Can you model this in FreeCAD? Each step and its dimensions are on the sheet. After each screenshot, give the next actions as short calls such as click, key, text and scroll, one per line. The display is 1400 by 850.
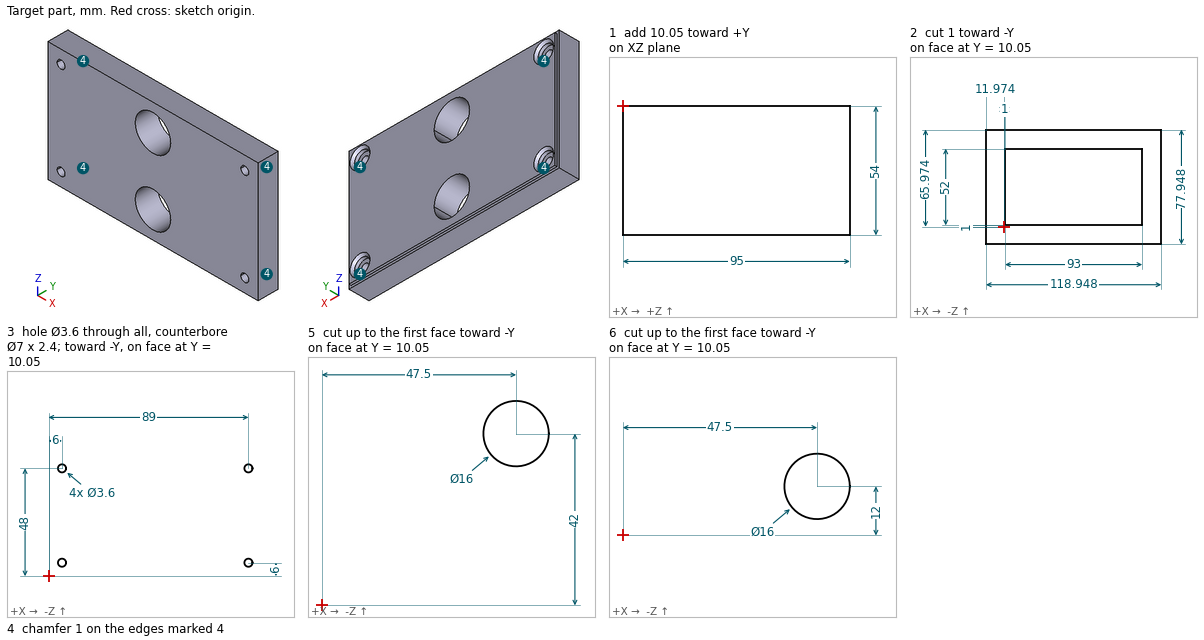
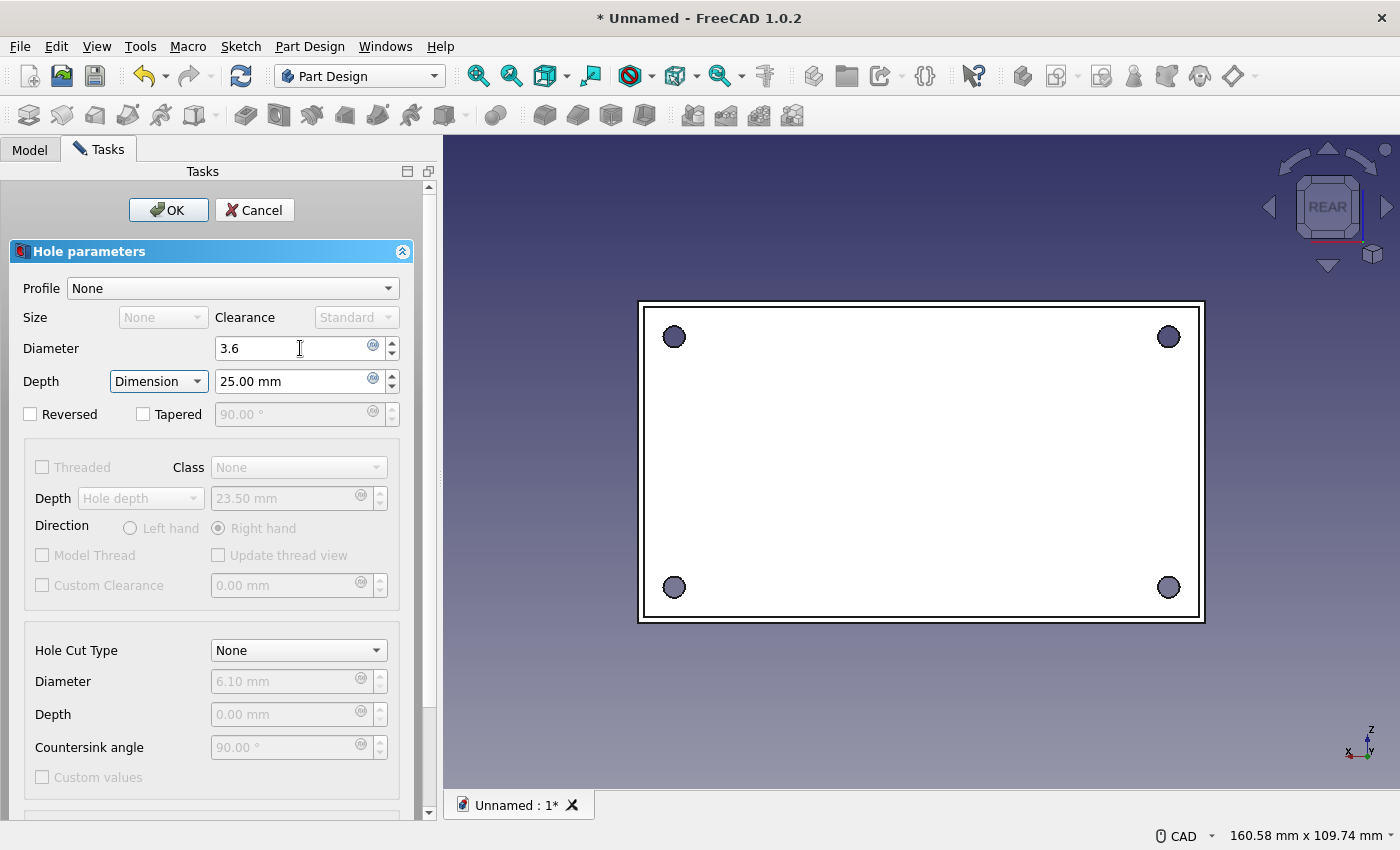
click(160, 382)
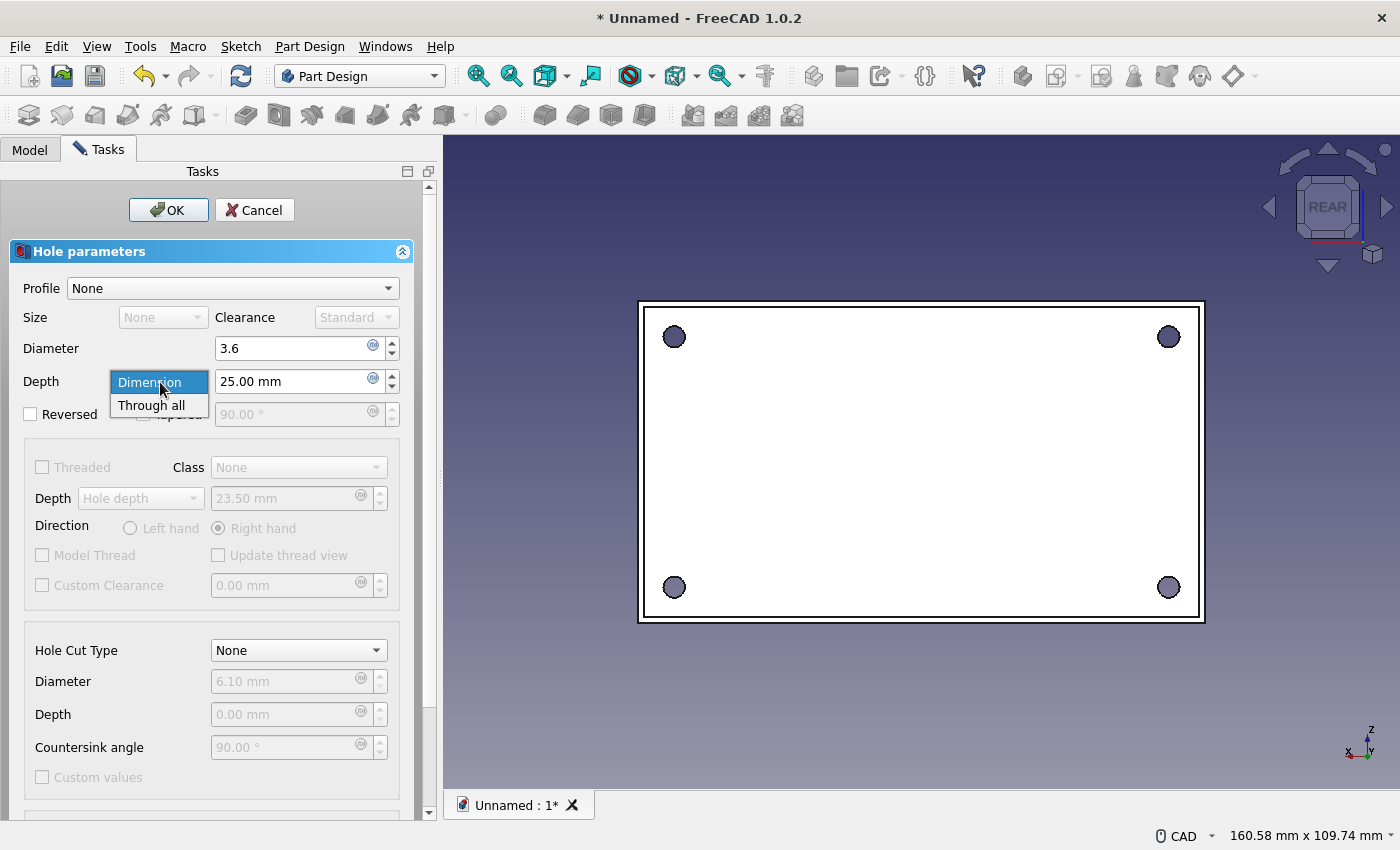
click(158, 406)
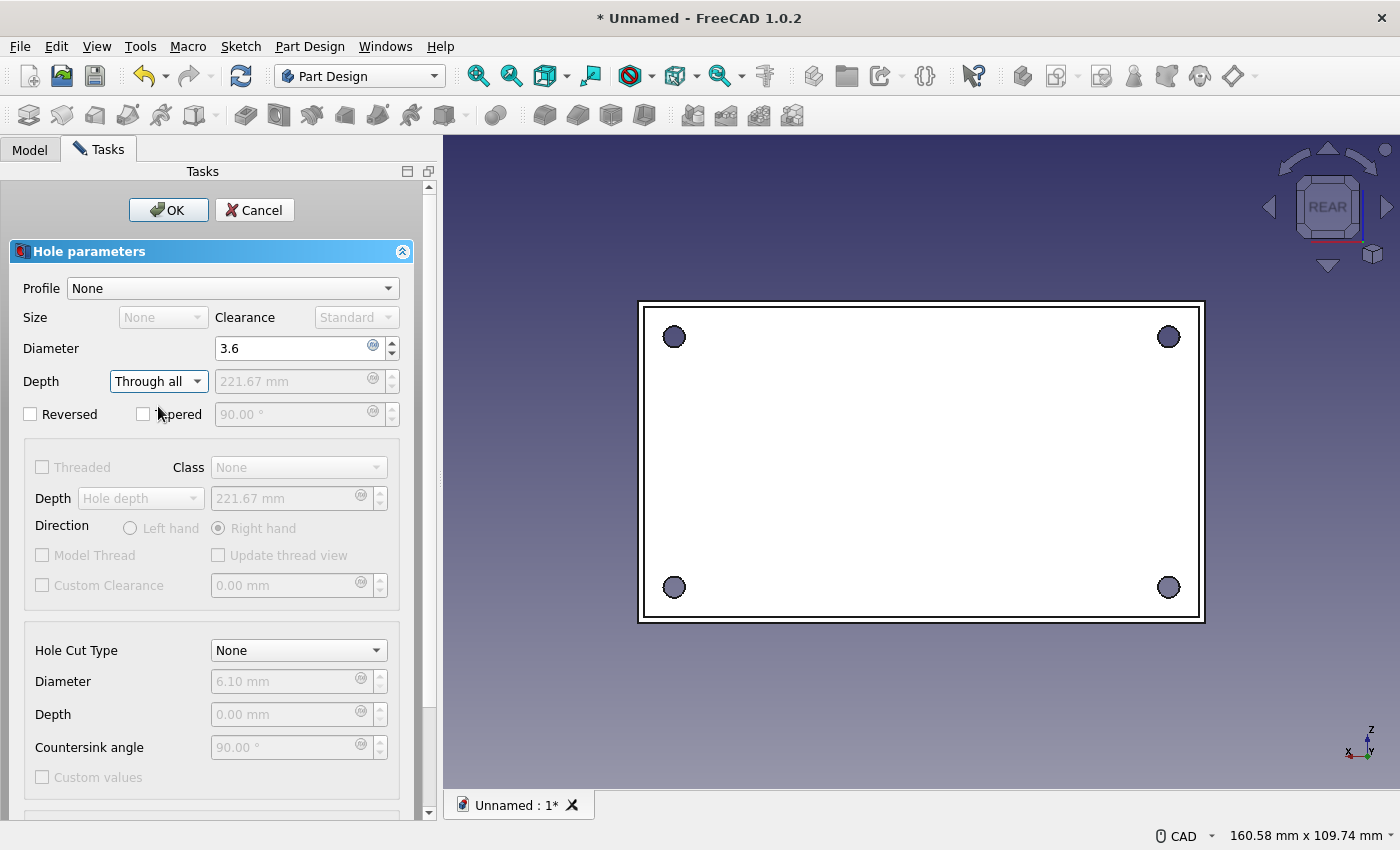
click(300, 650)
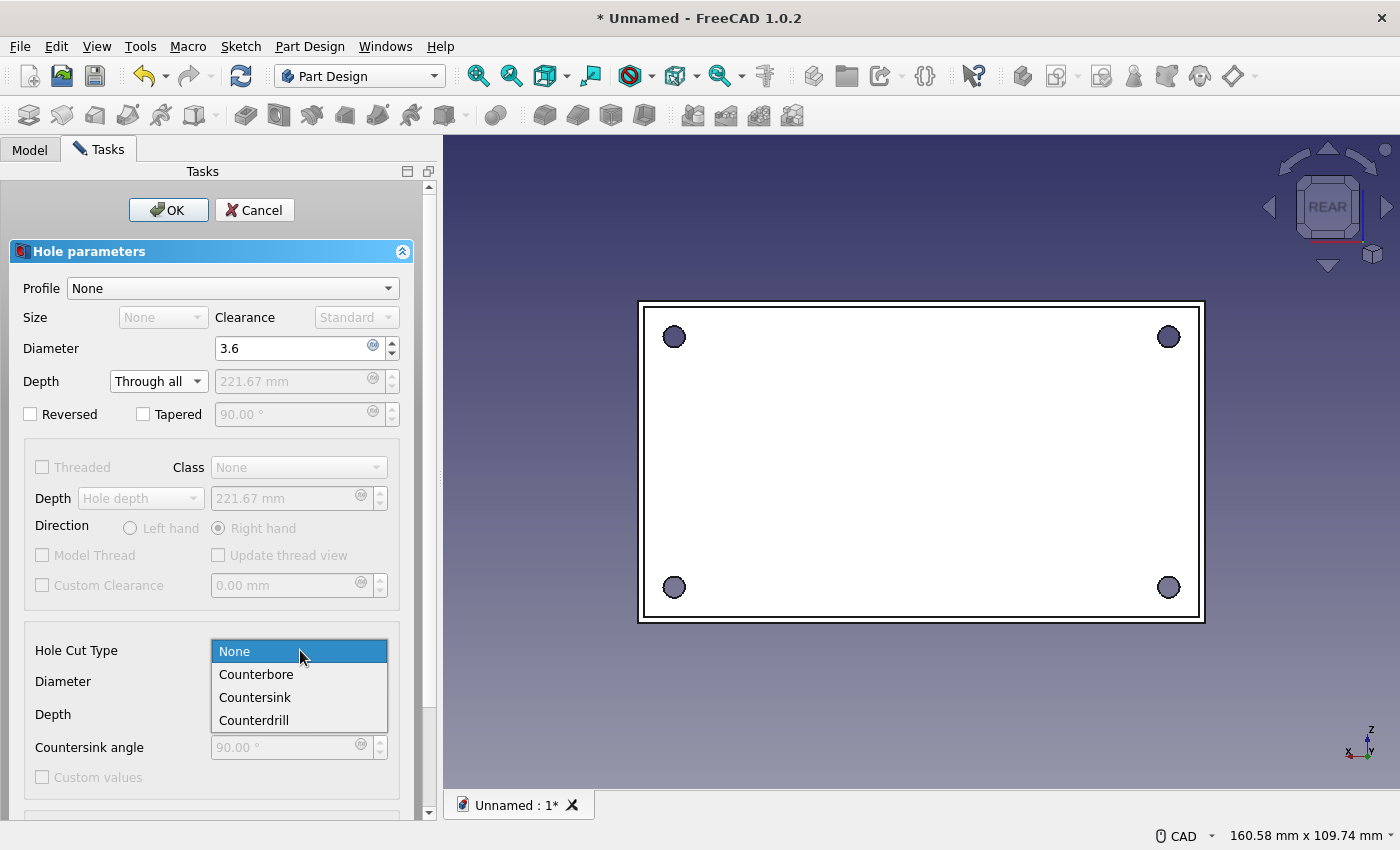
click(298, 674)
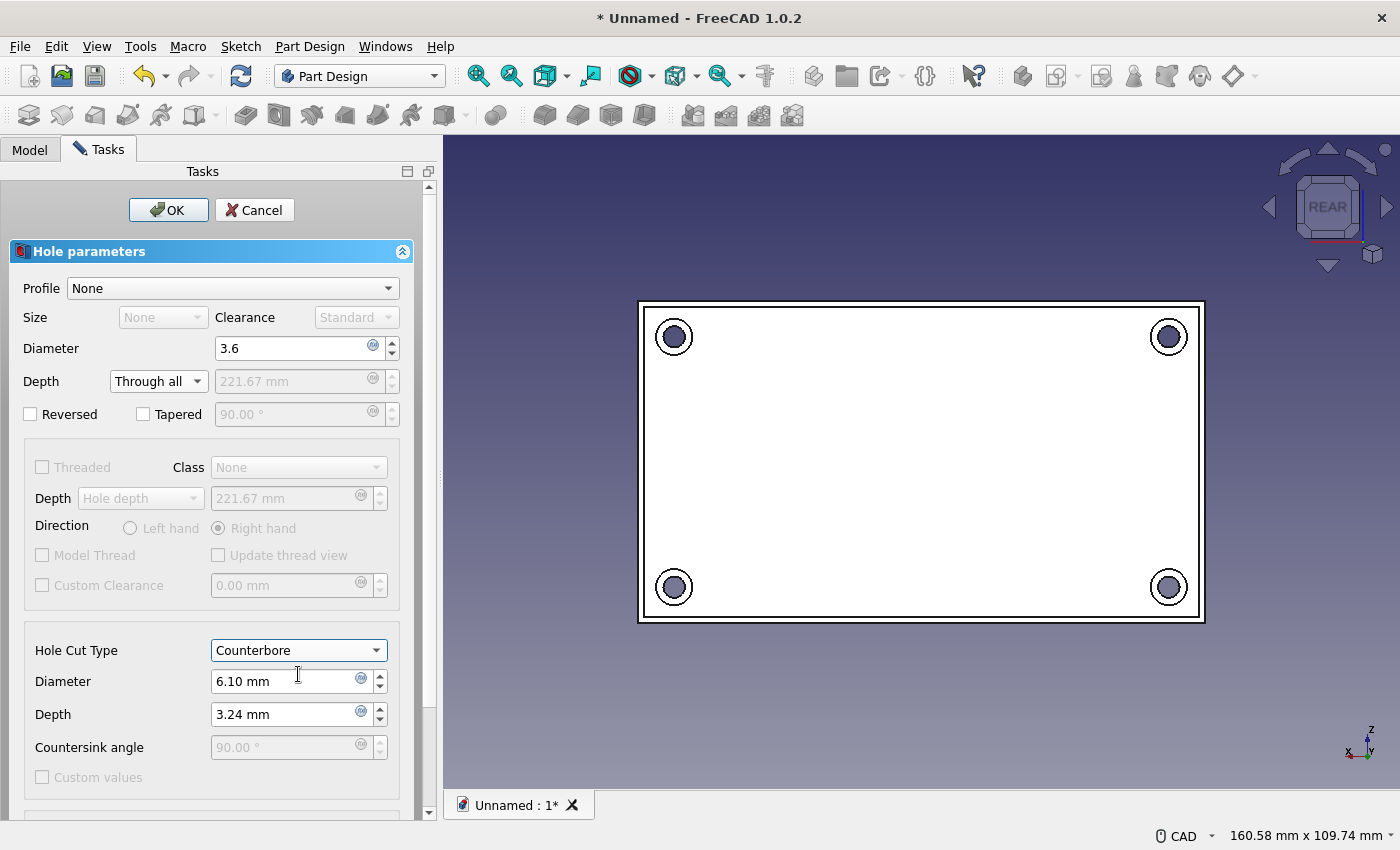
triple_click(292, 682)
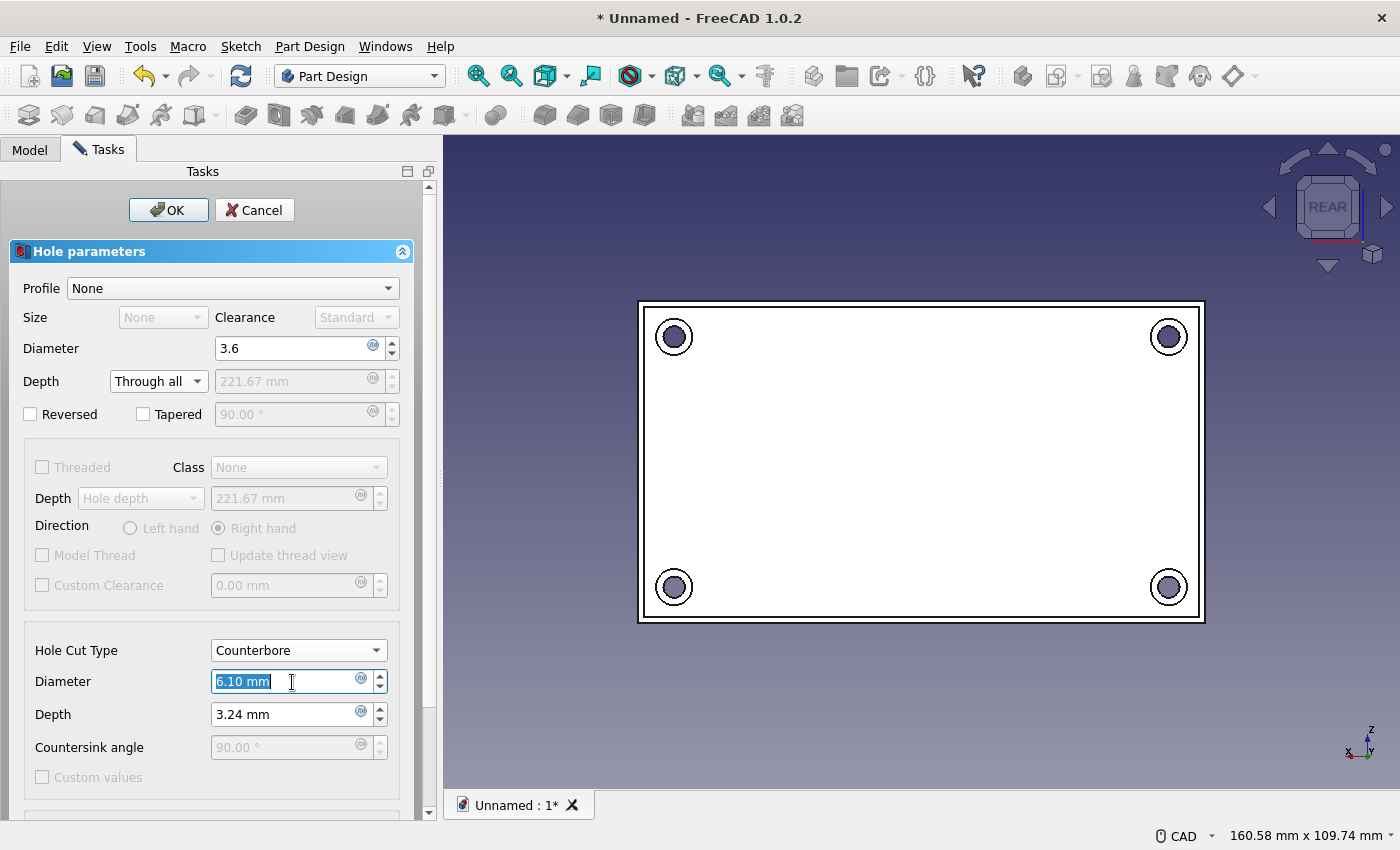
text(7)
key(Tab)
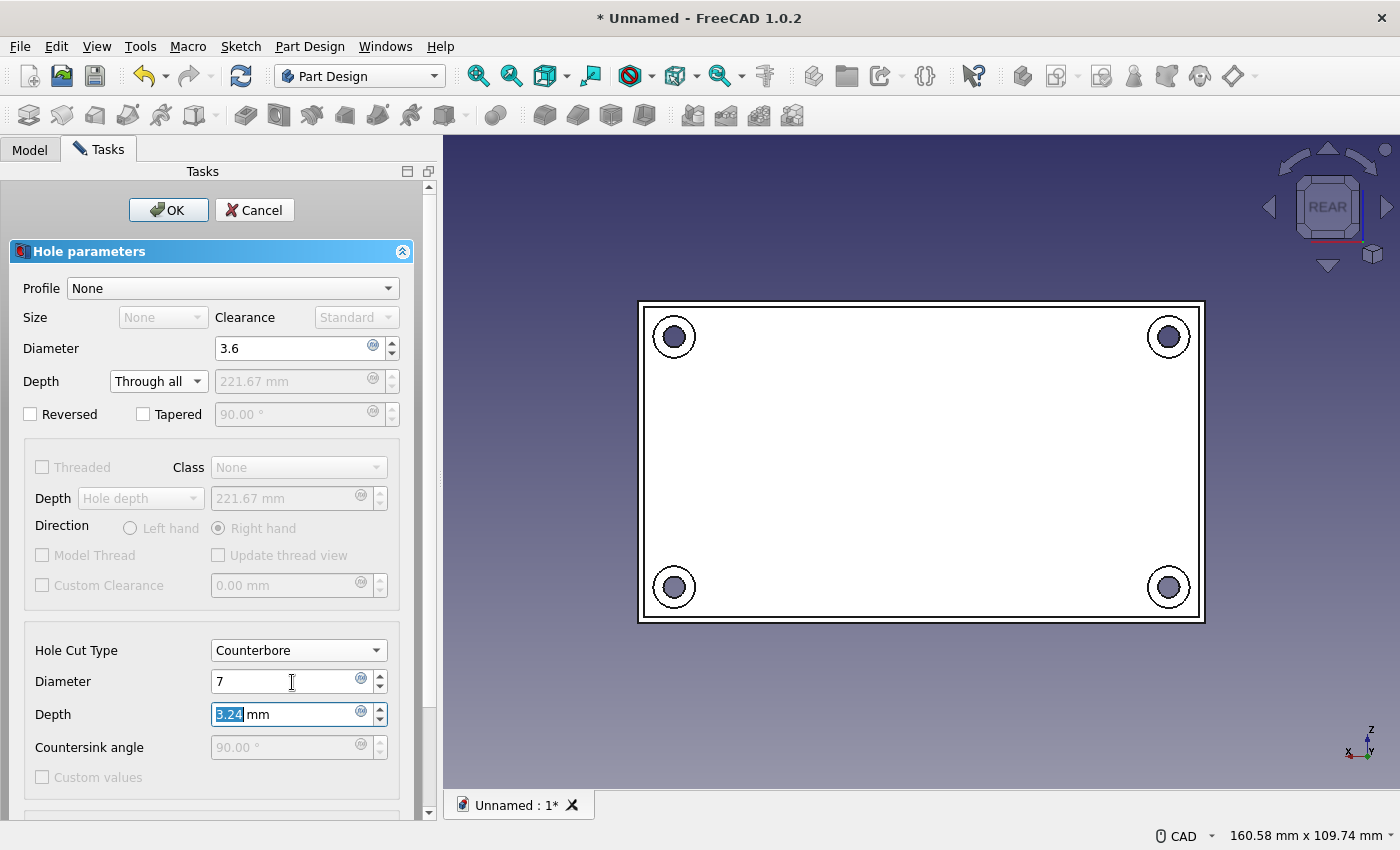
text(2.4)
key(Tab)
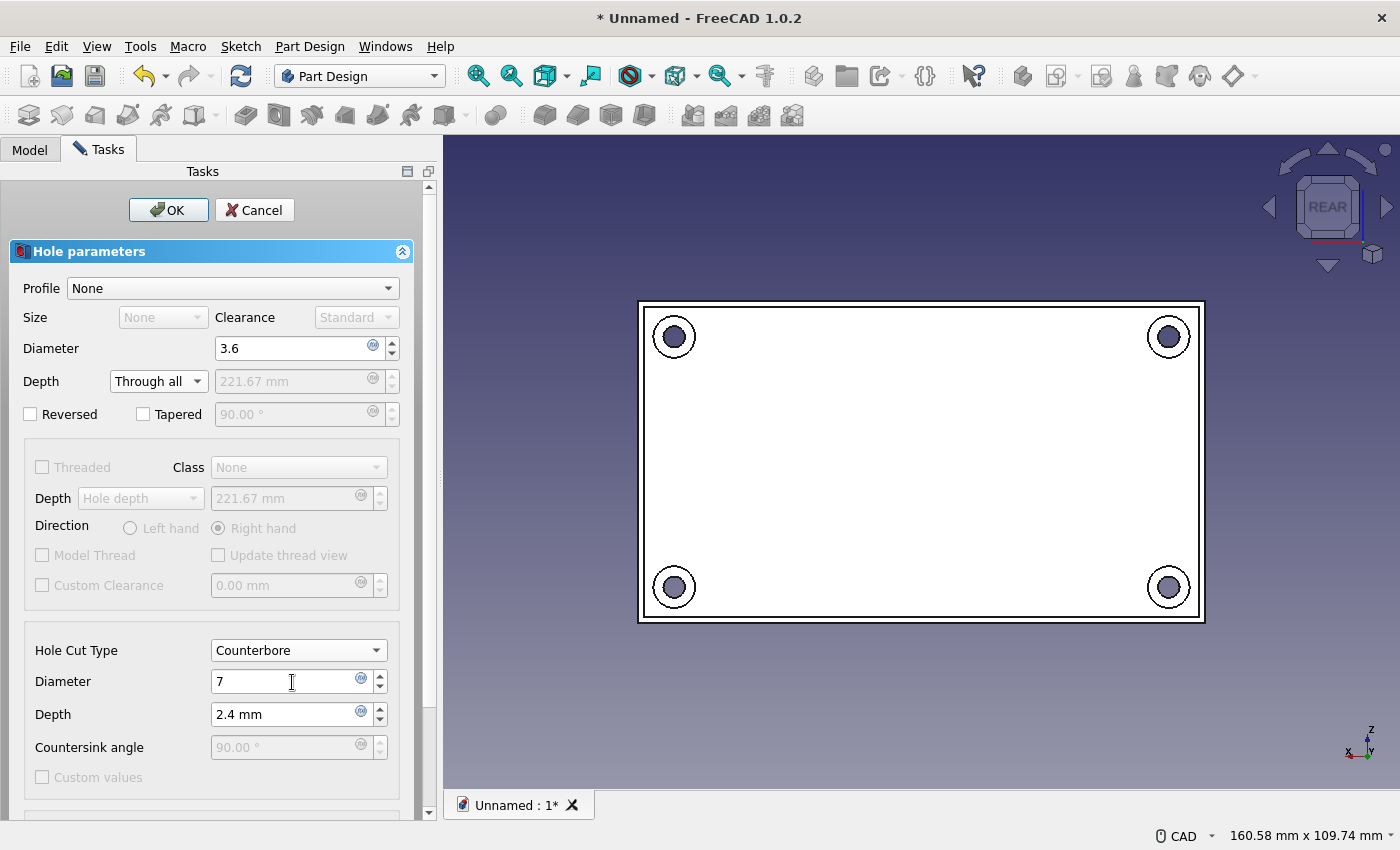
click(169, 210)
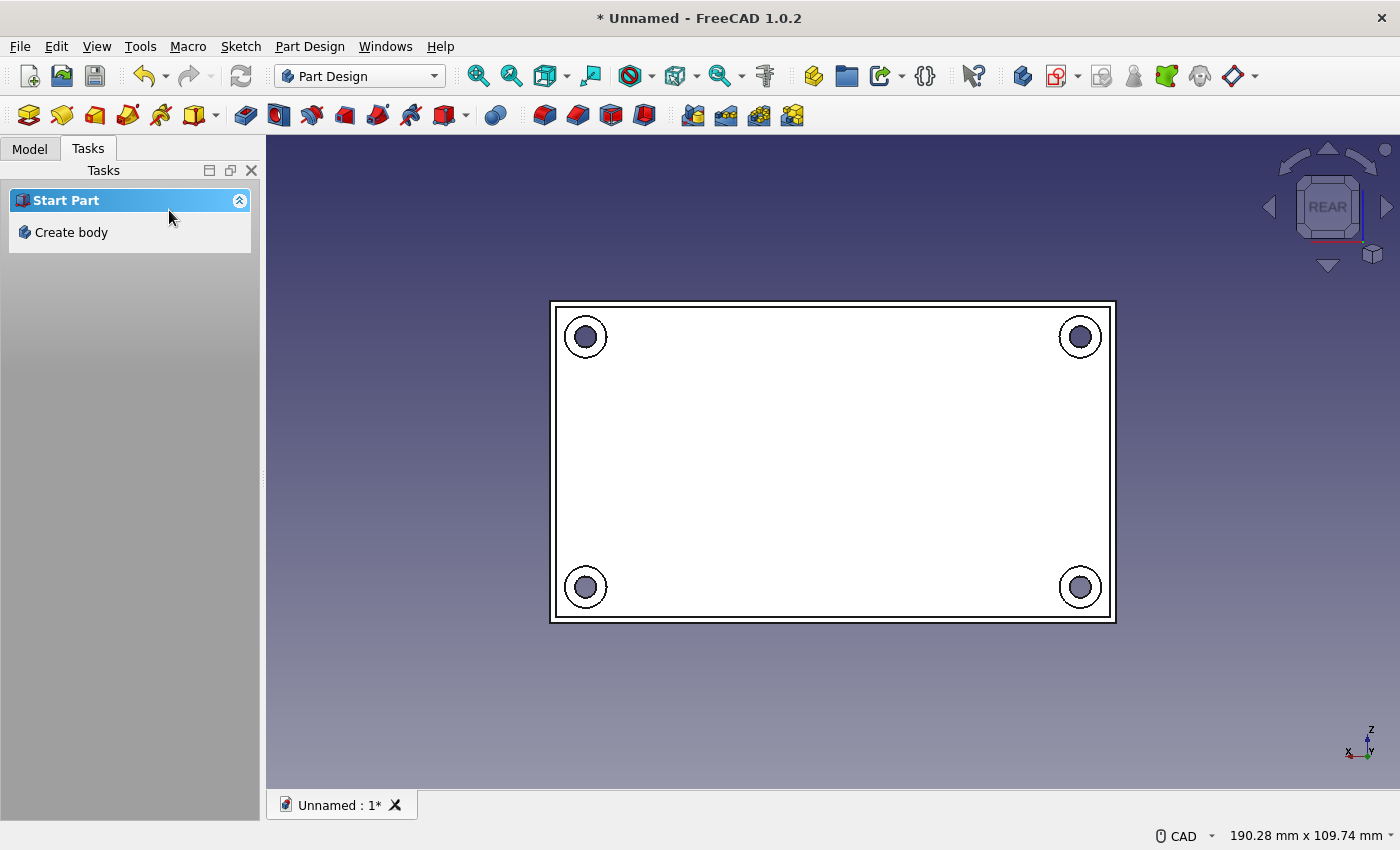
click(1059, 336)